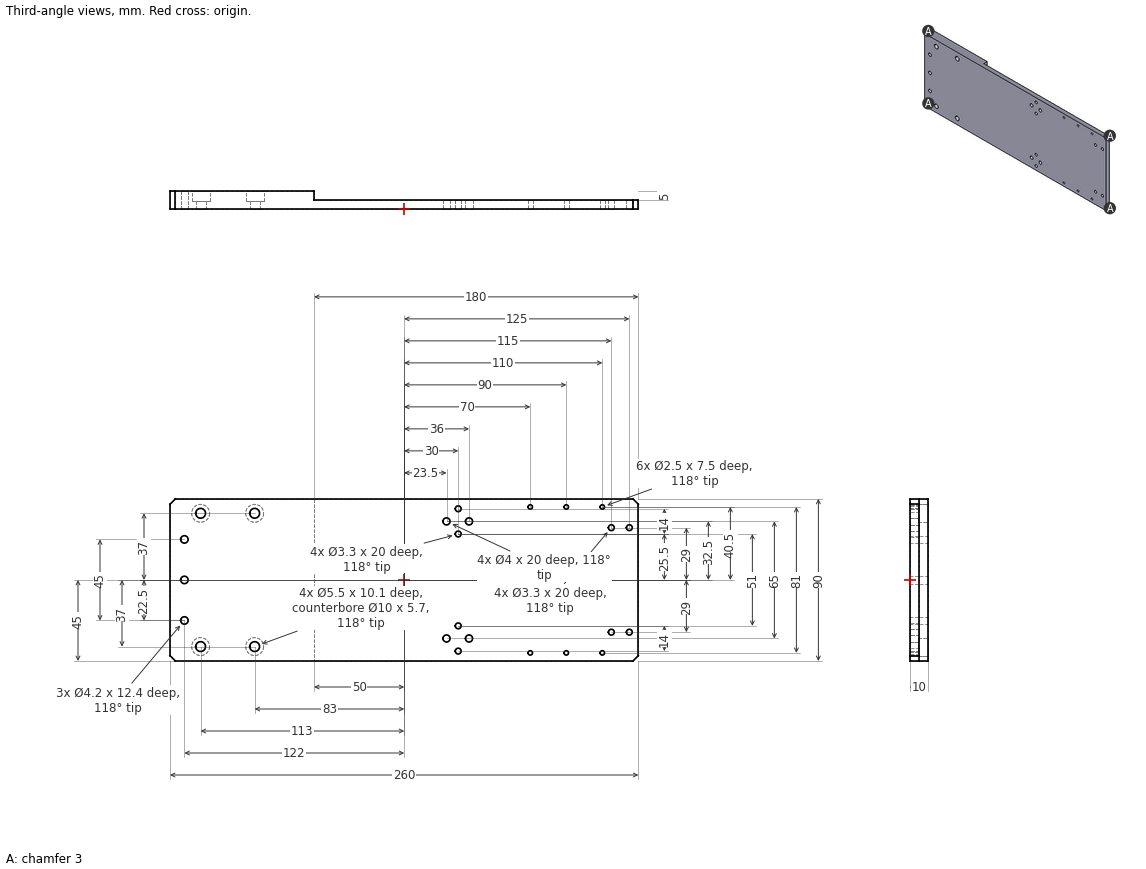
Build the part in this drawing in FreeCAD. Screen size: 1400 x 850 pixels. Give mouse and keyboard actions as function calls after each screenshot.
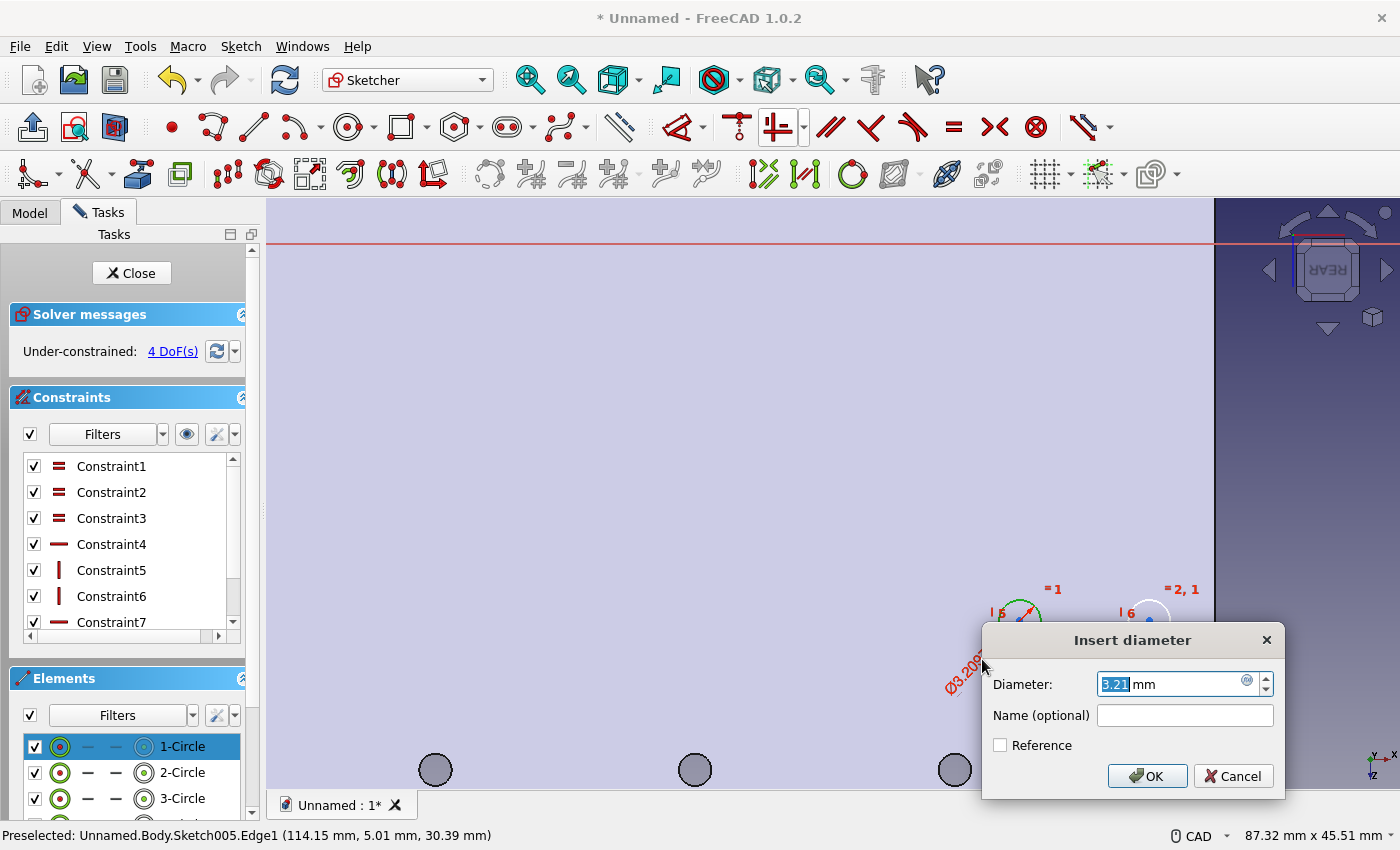
text(3.3)
key(Return)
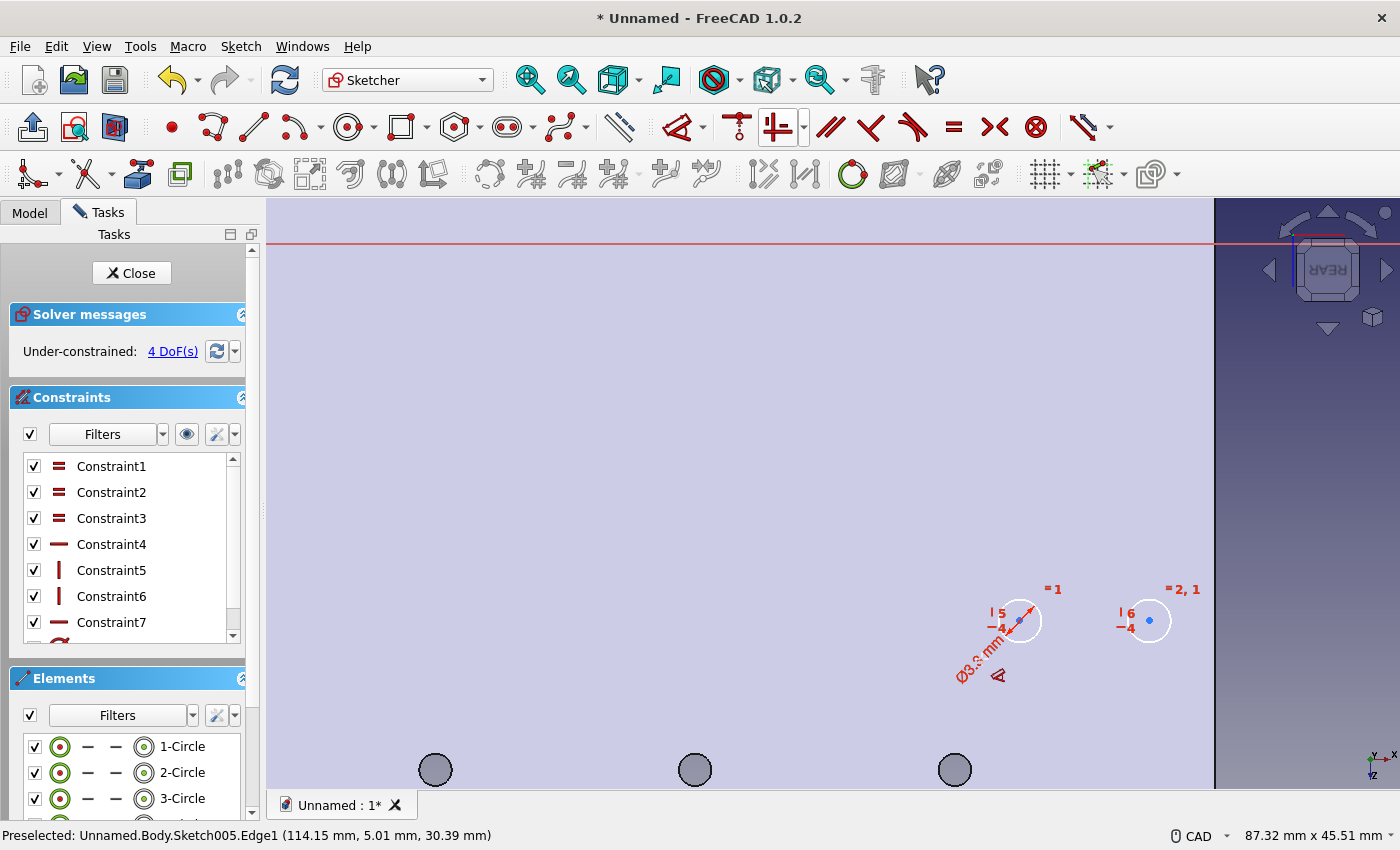
click(1020, 621)
click(1054, 432)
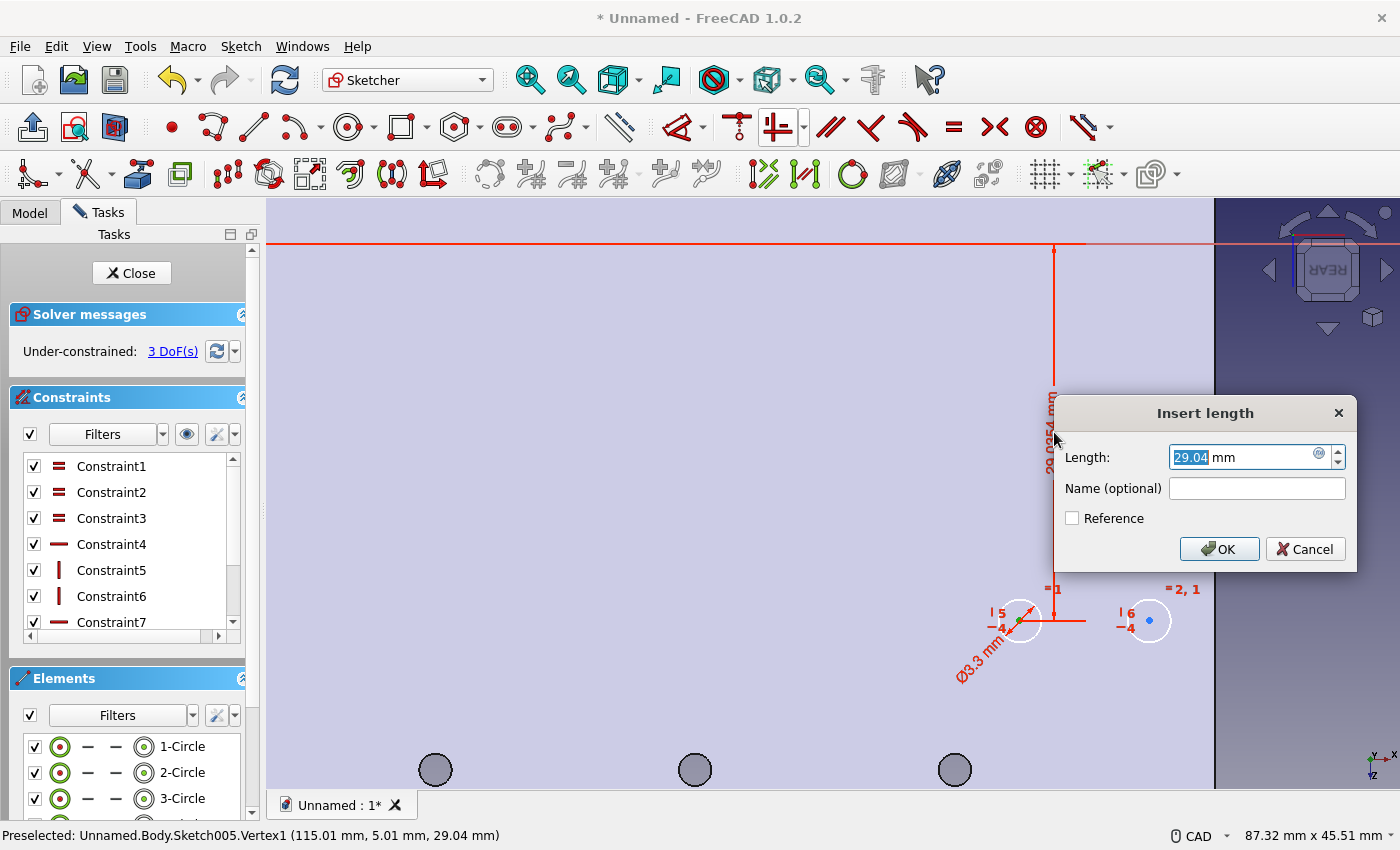
text(29)
key(Return)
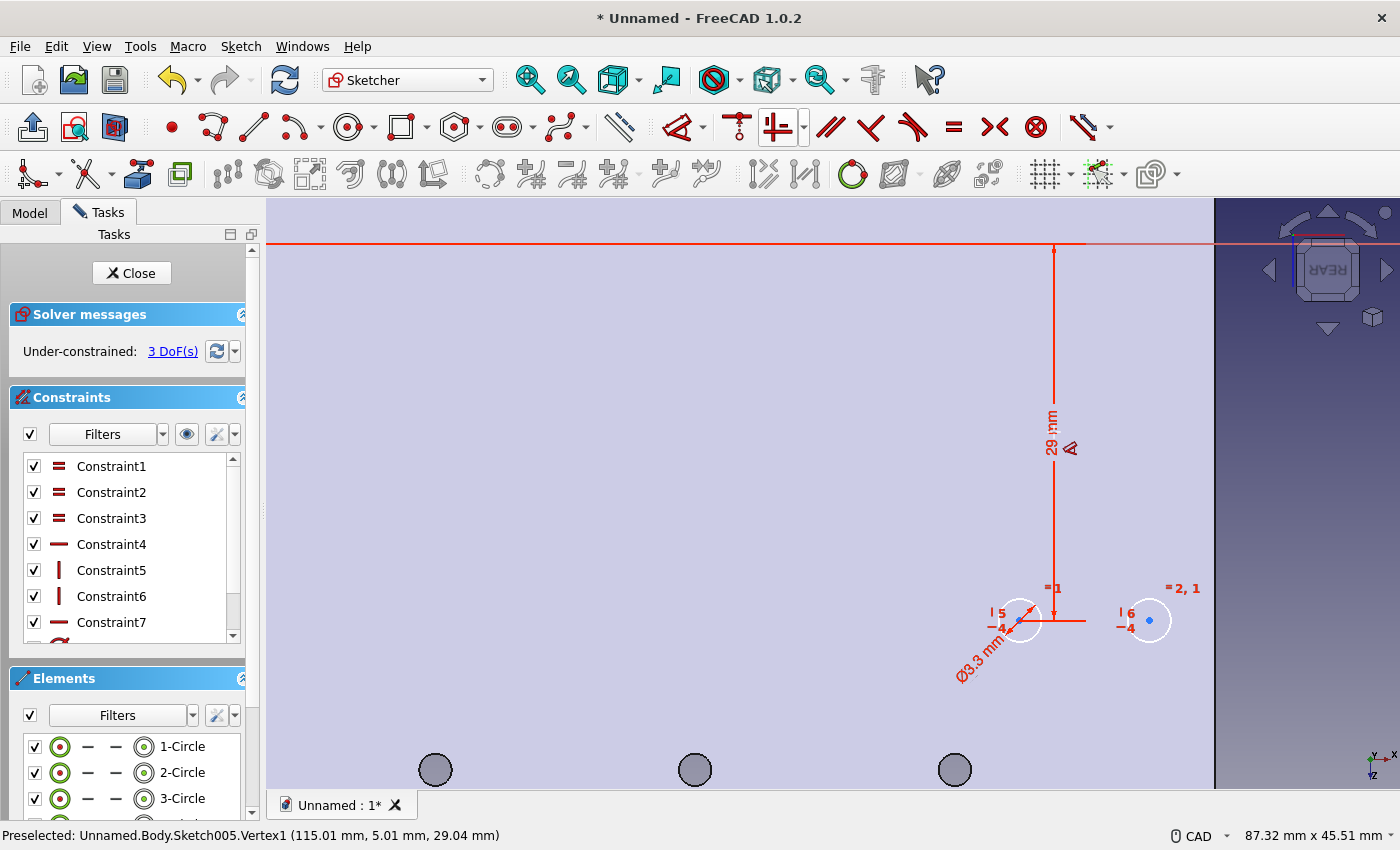
scroll(1006, 639, down, 5)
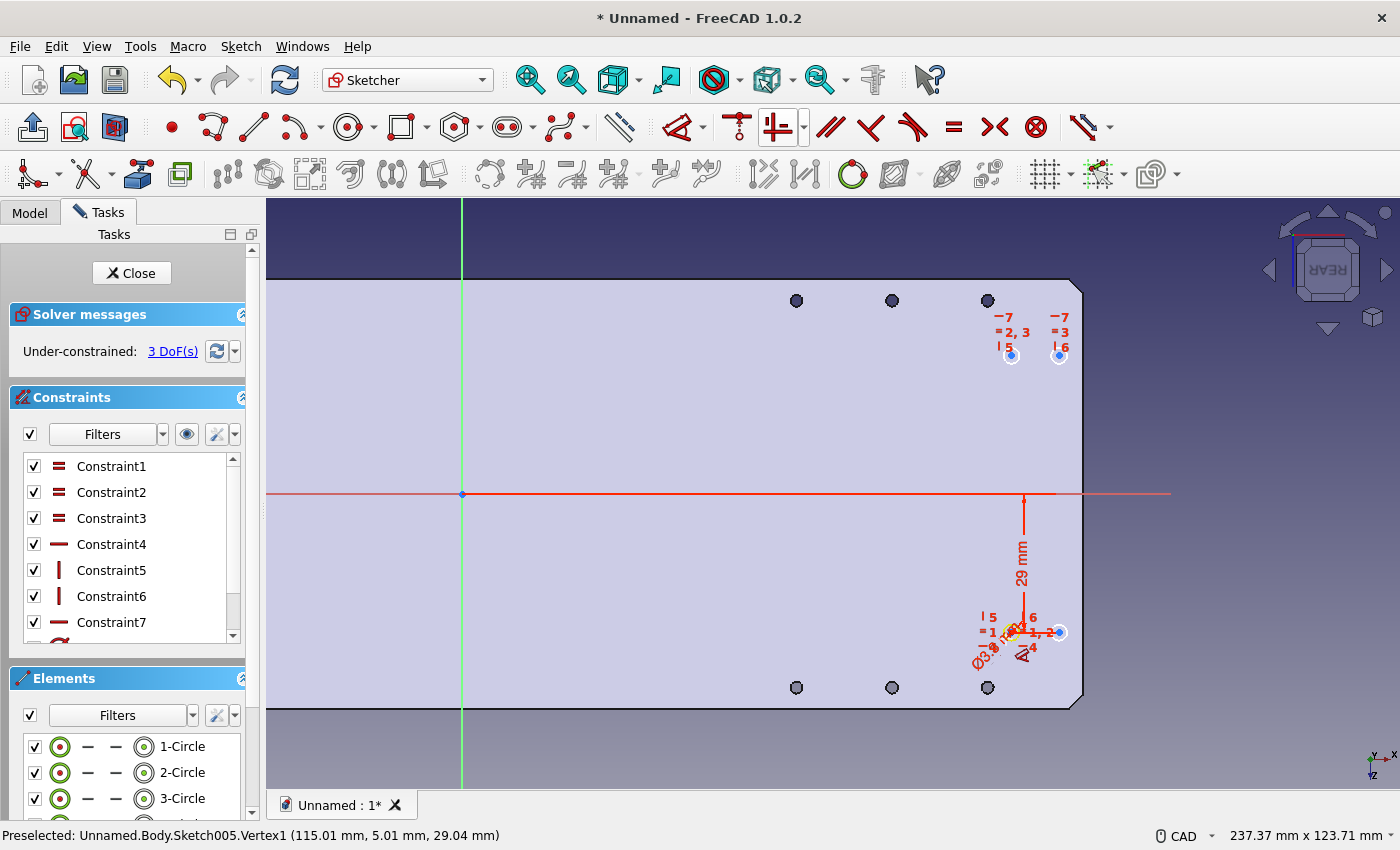
click(1012, 356)
click(428, 425)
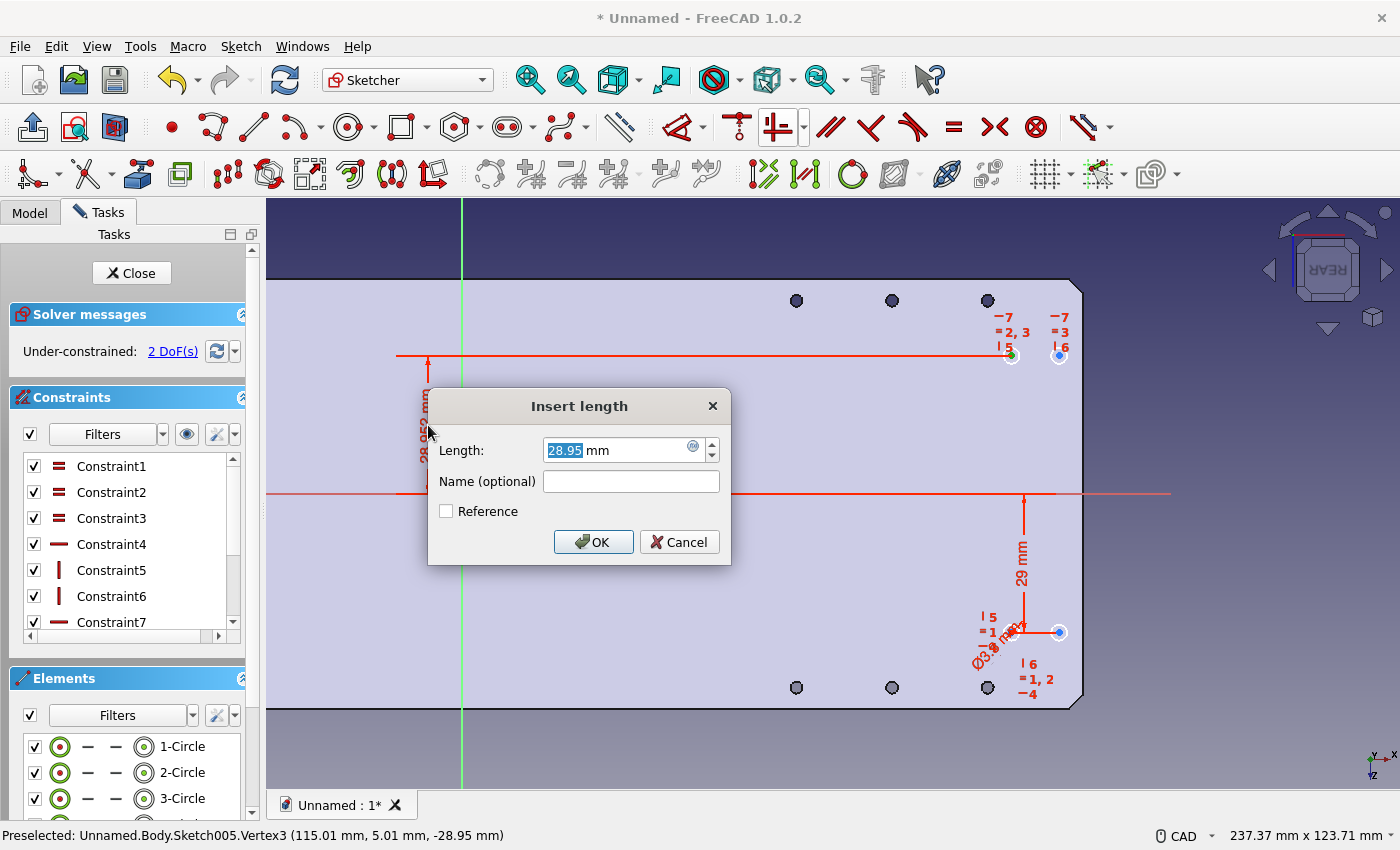
text(29)
key(Return)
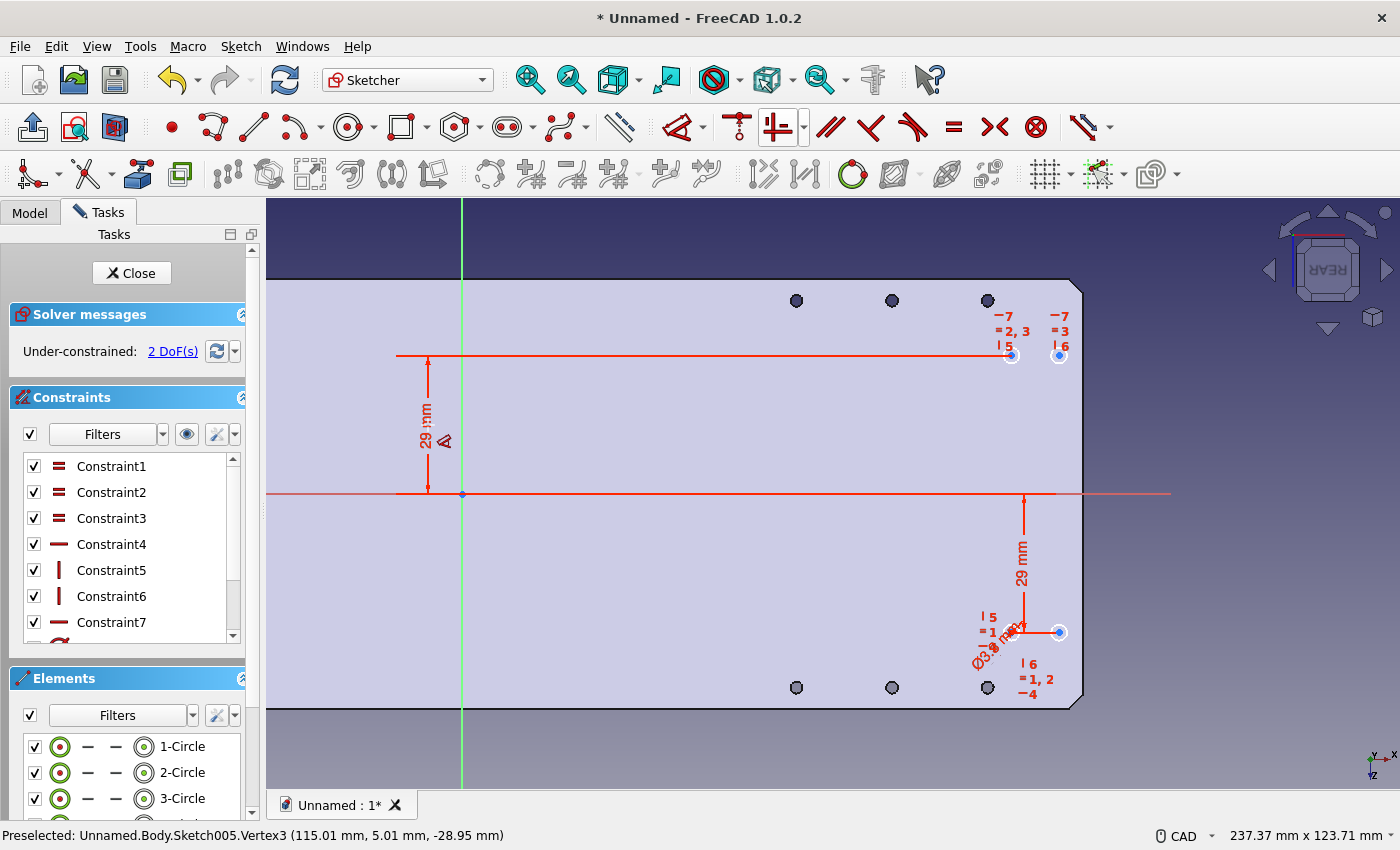
click(1012, 633)
click(737, 667)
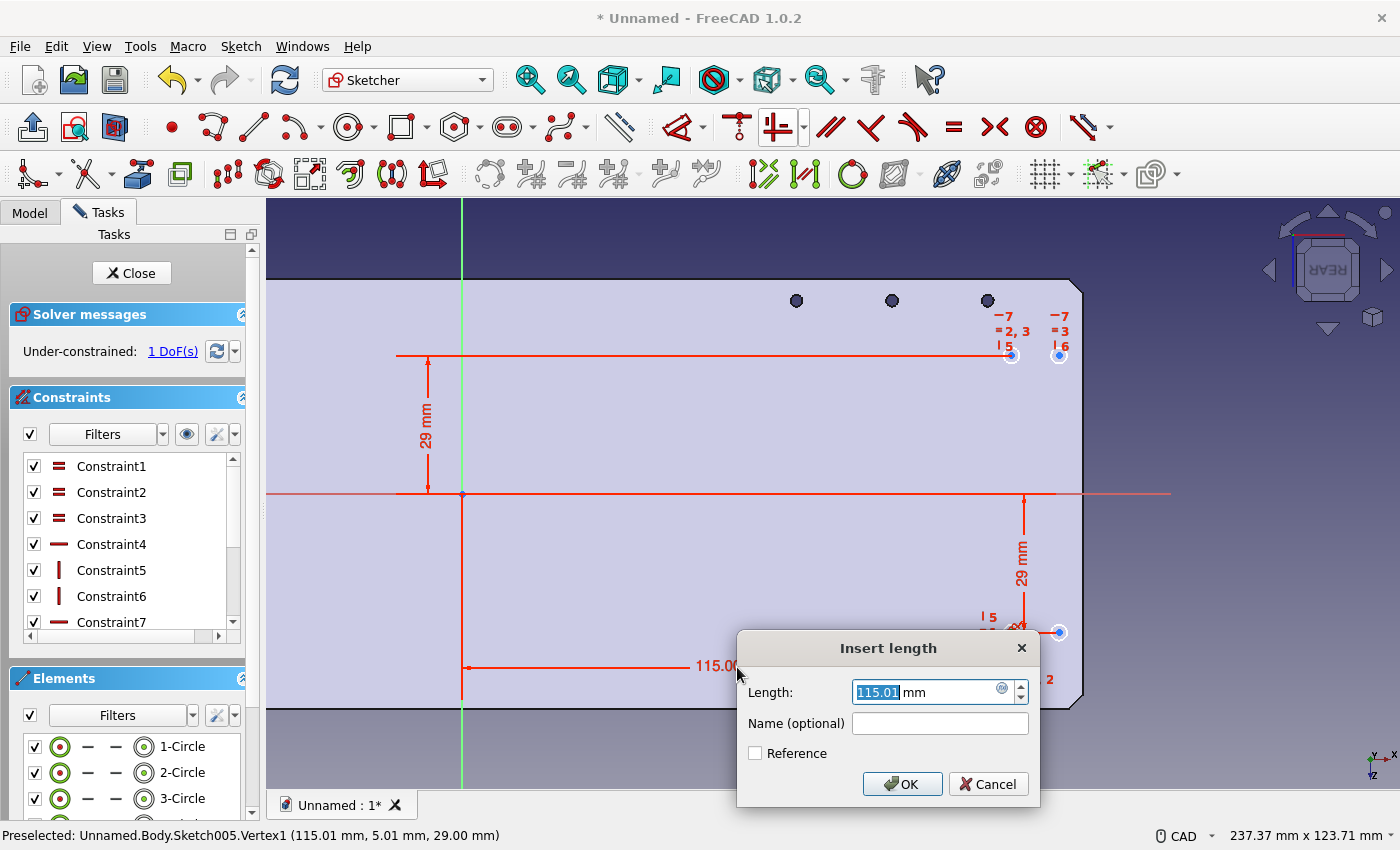
text(115)
key(Return)